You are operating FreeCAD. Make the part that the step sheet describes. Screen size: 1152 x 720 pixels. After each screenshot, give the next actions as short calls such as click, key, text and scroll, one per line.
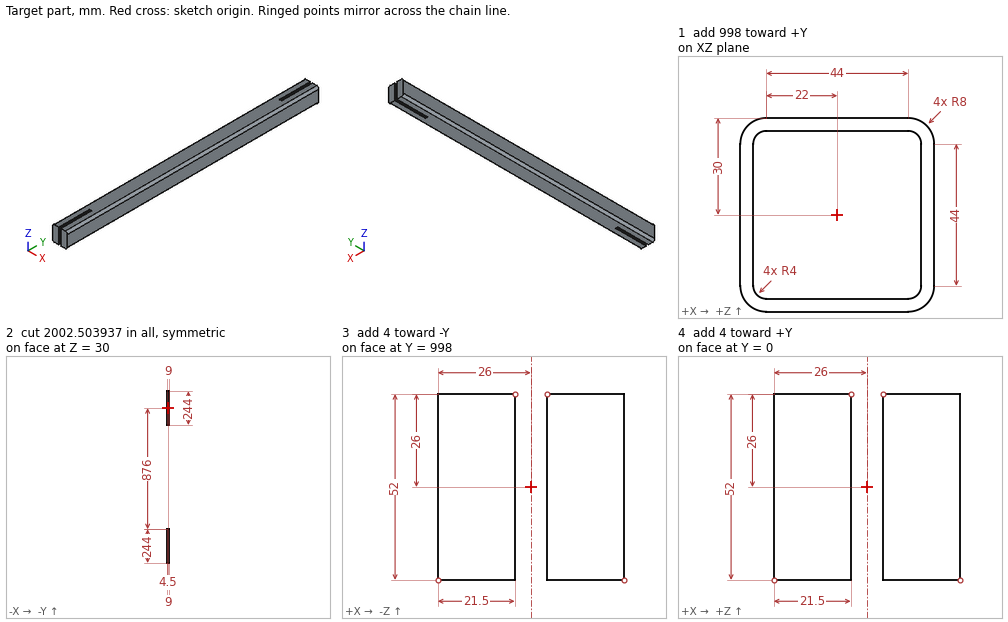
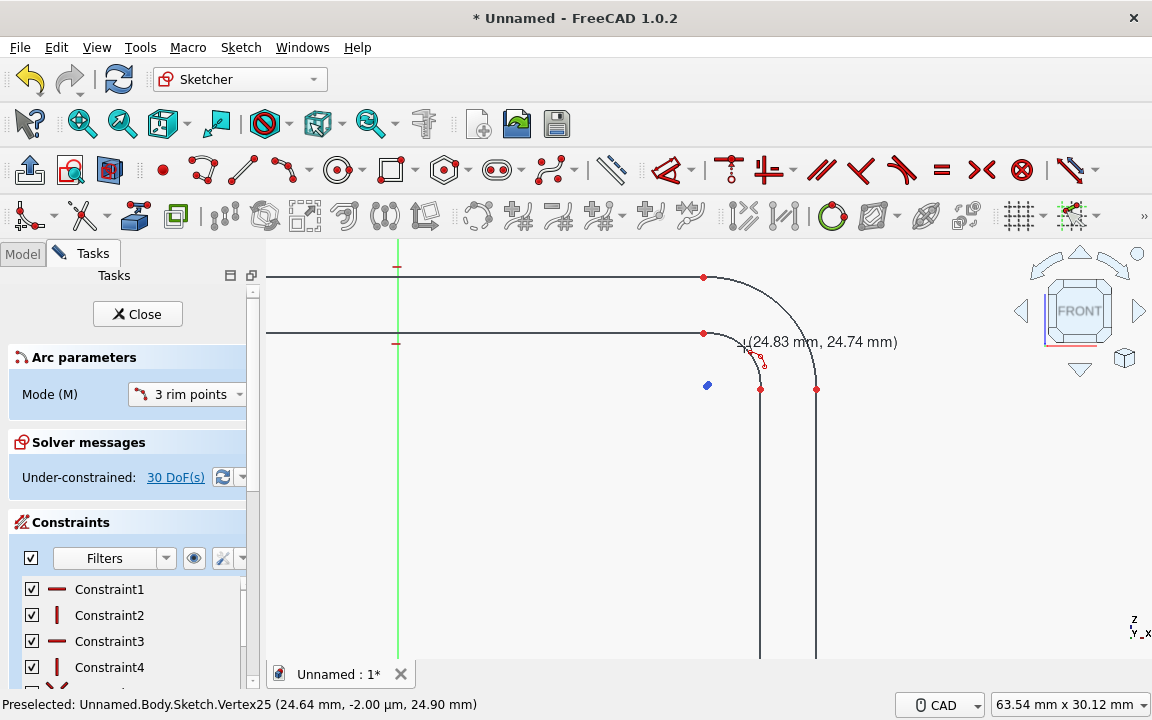
scroll(745, 344, down, 6)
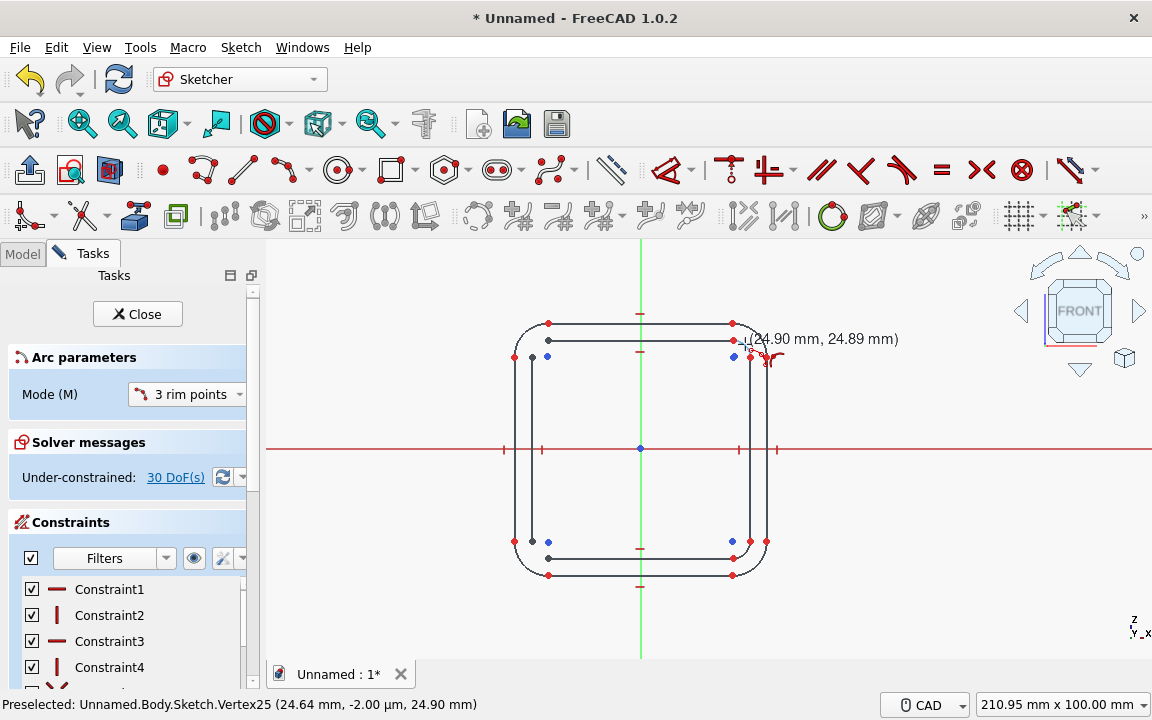
click(548, 341)
click(532, 358)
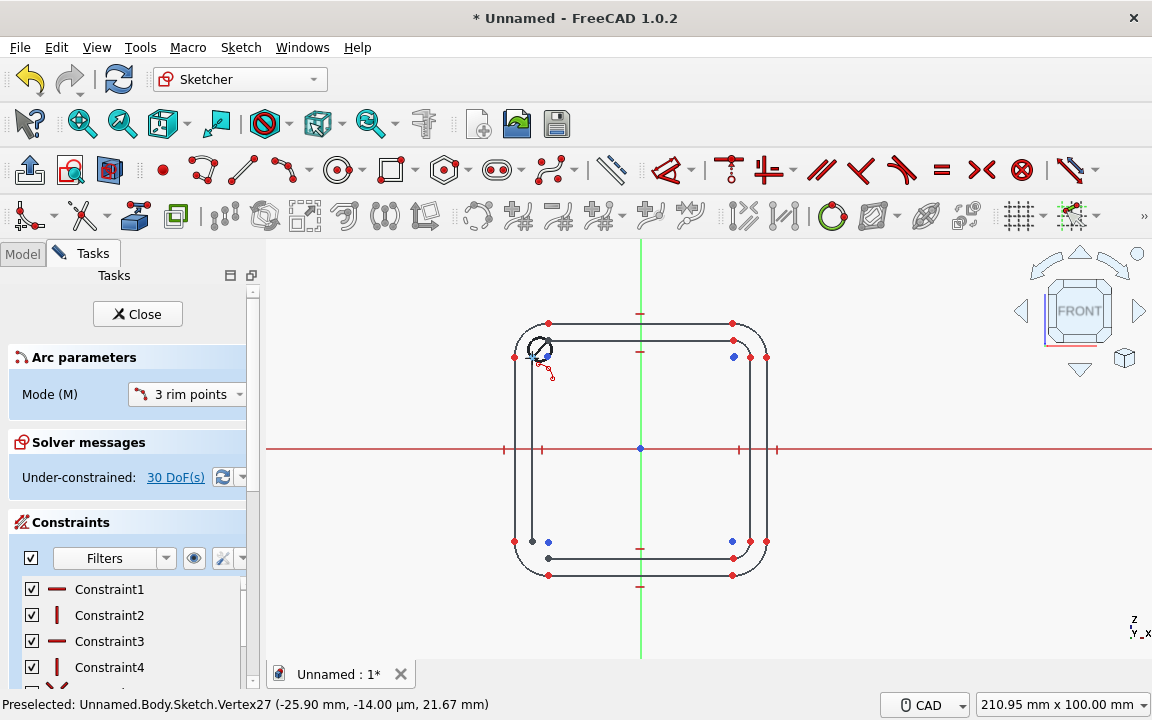
scroll(537, 345, up, 6)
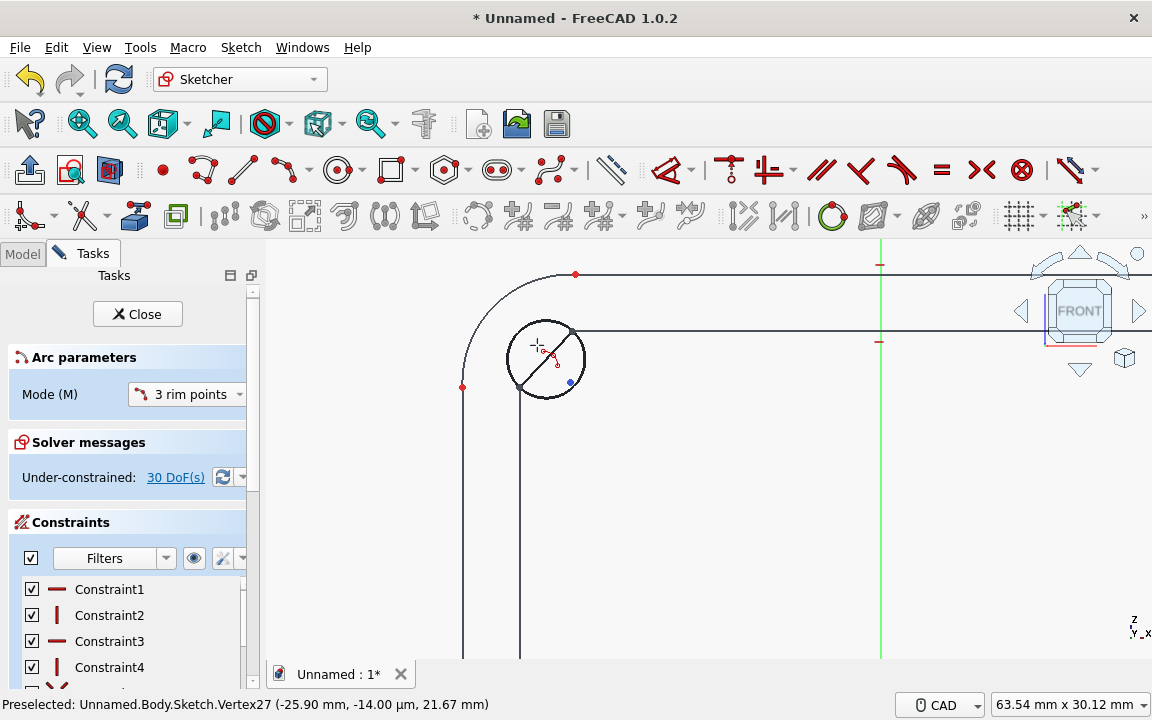
click(535, 343)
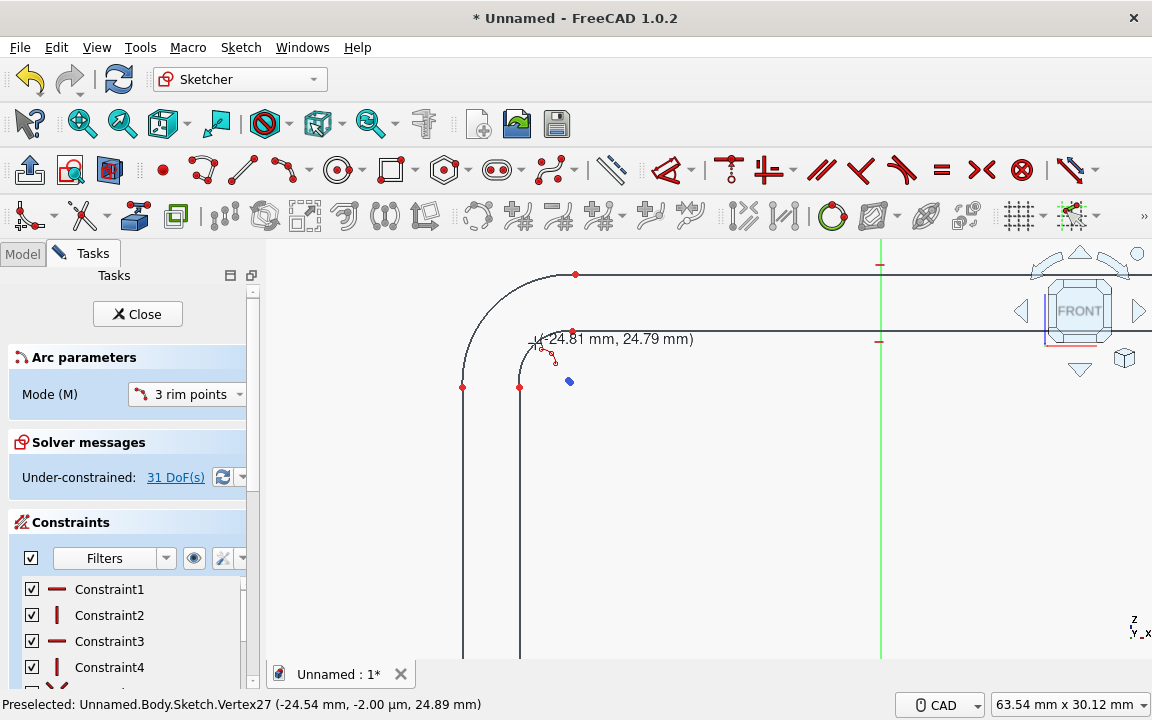
scroll(537, 345, down, 6)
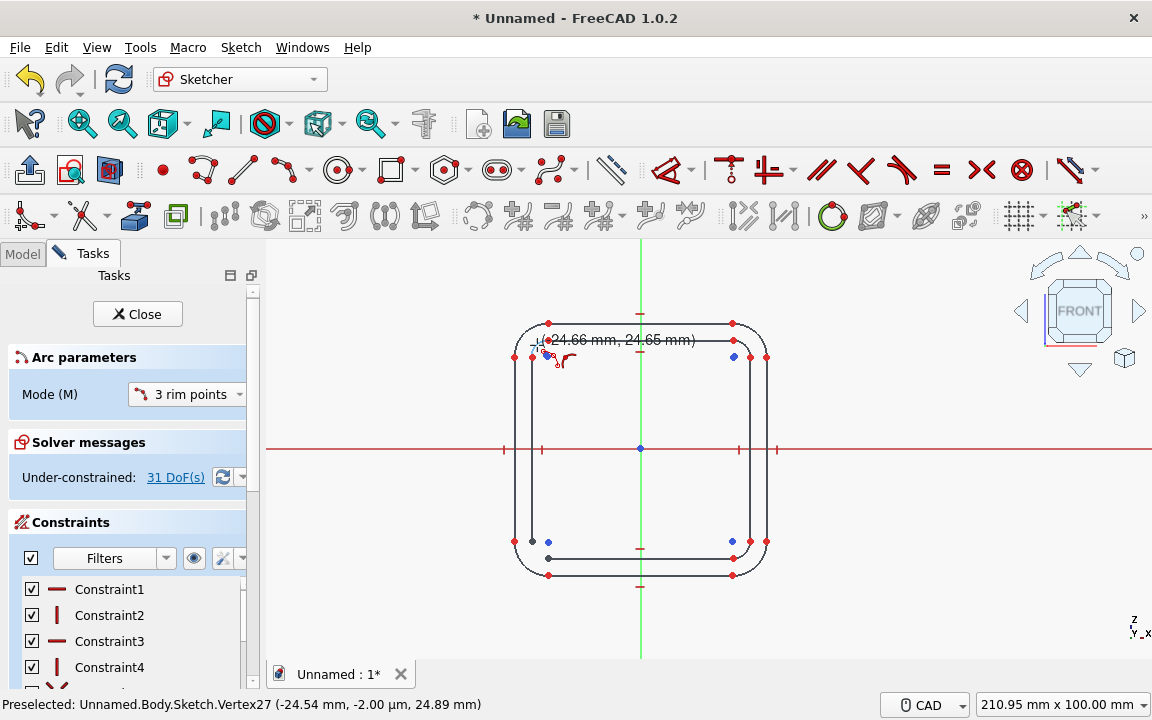
click(532, 542)
click(548, 559)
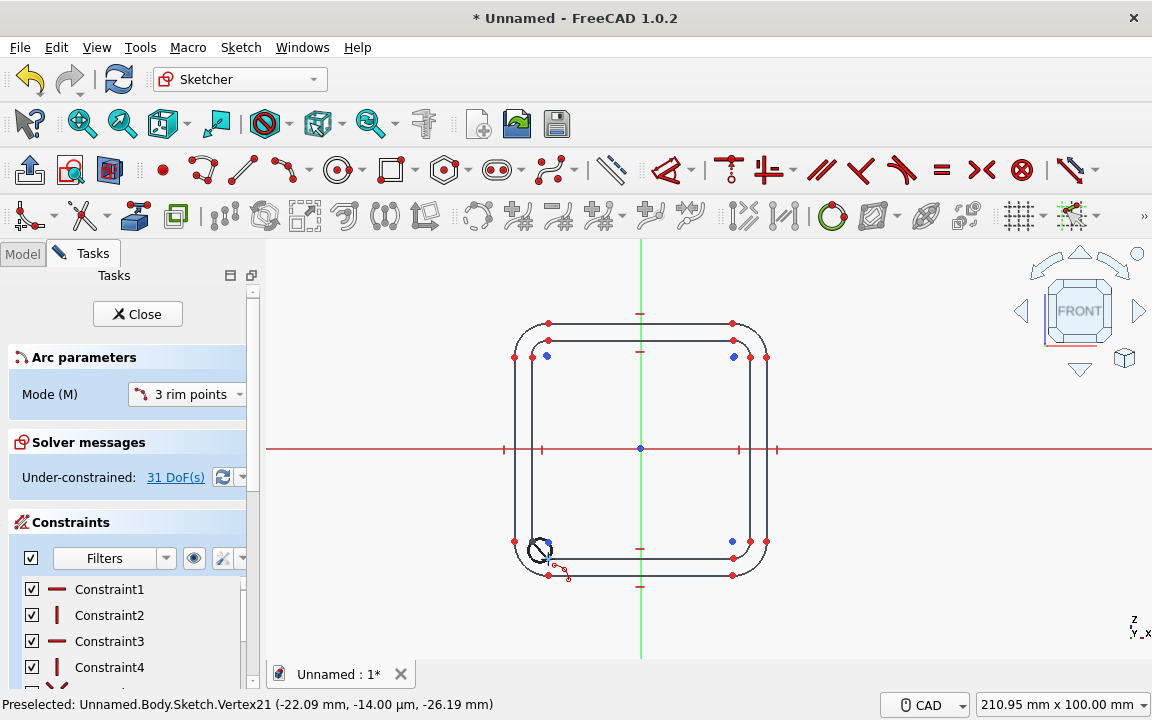
scroll(537, 553, up, 6)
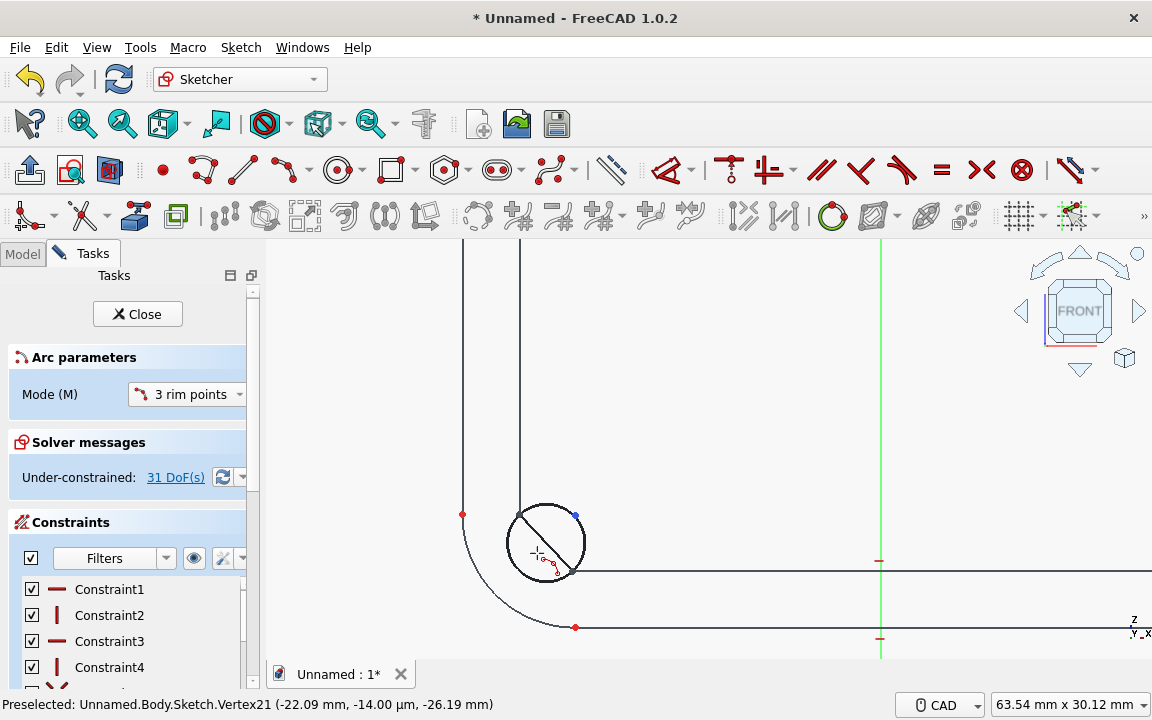
click(535, 552)
key(Escape)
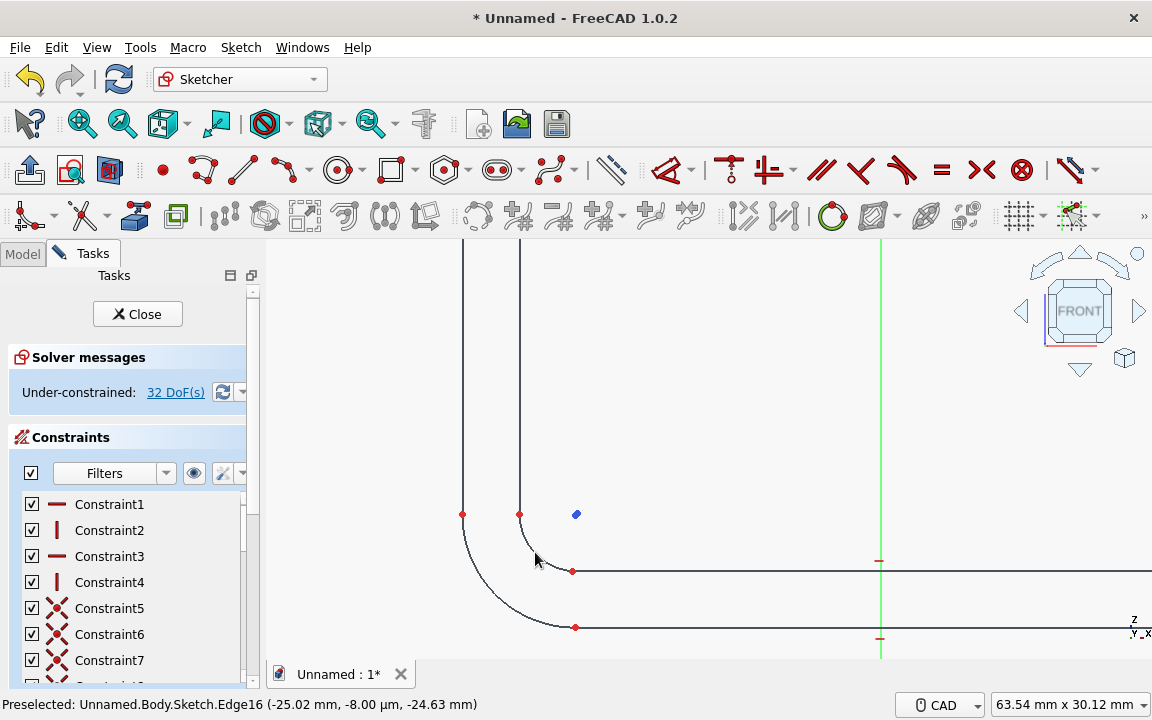
scroll(537, 554, down, 6)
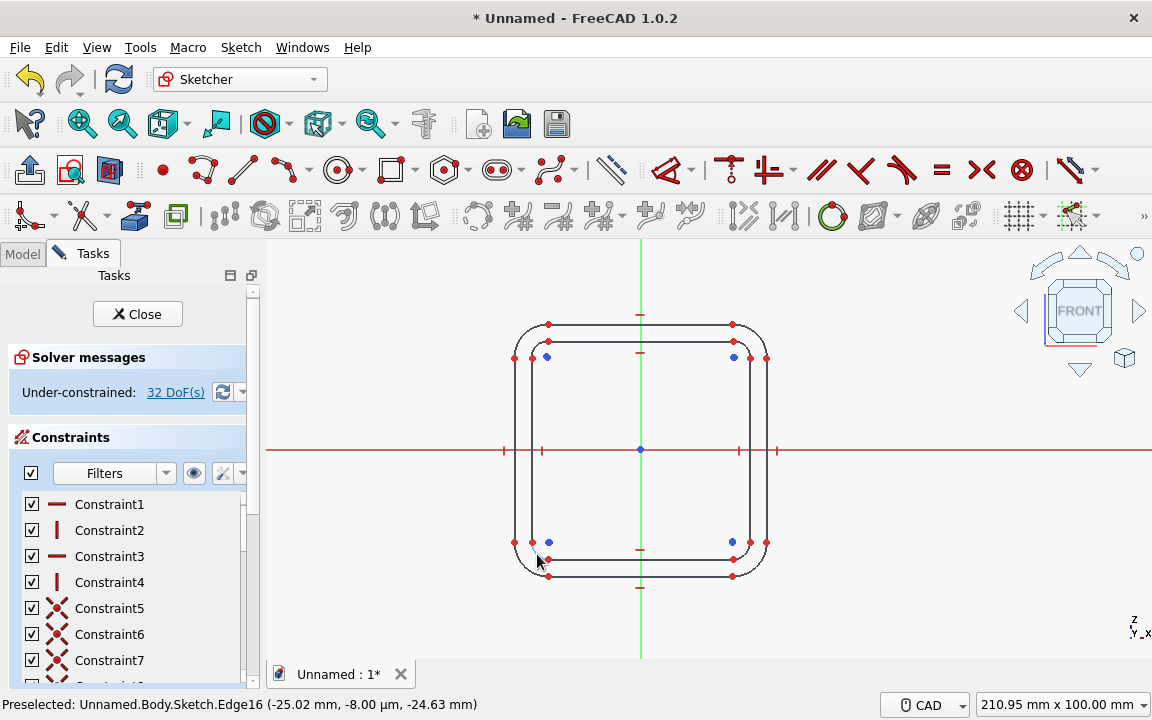
click(604, 325)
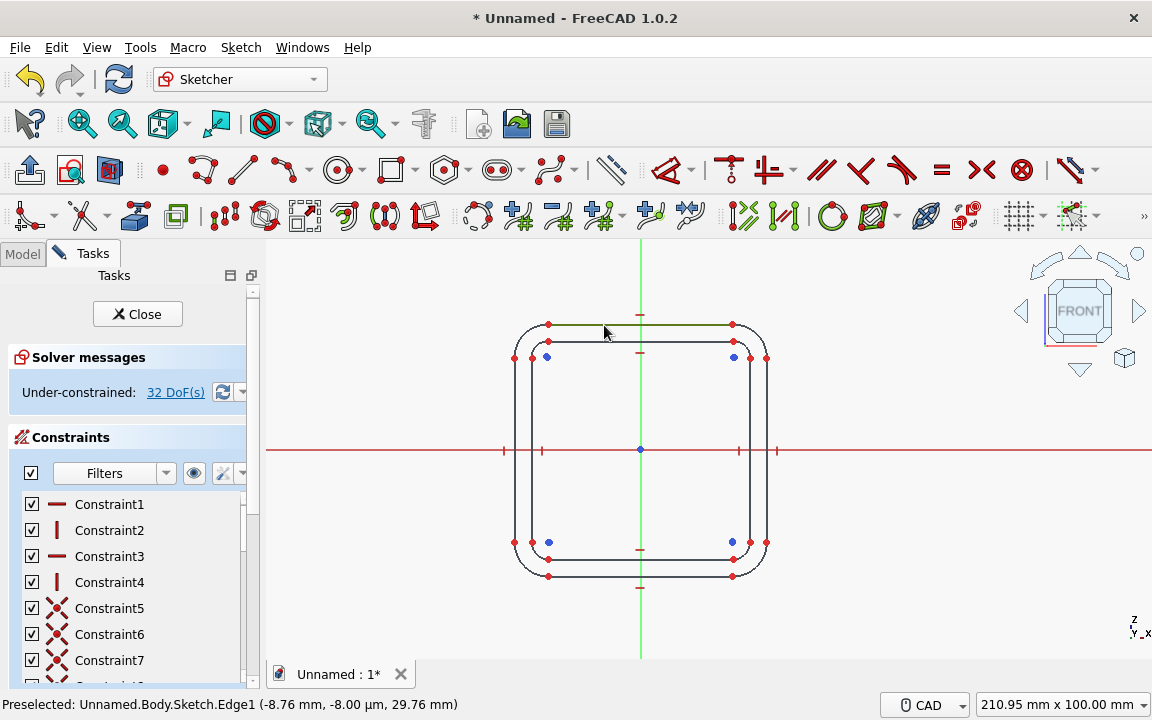
click(763, 343)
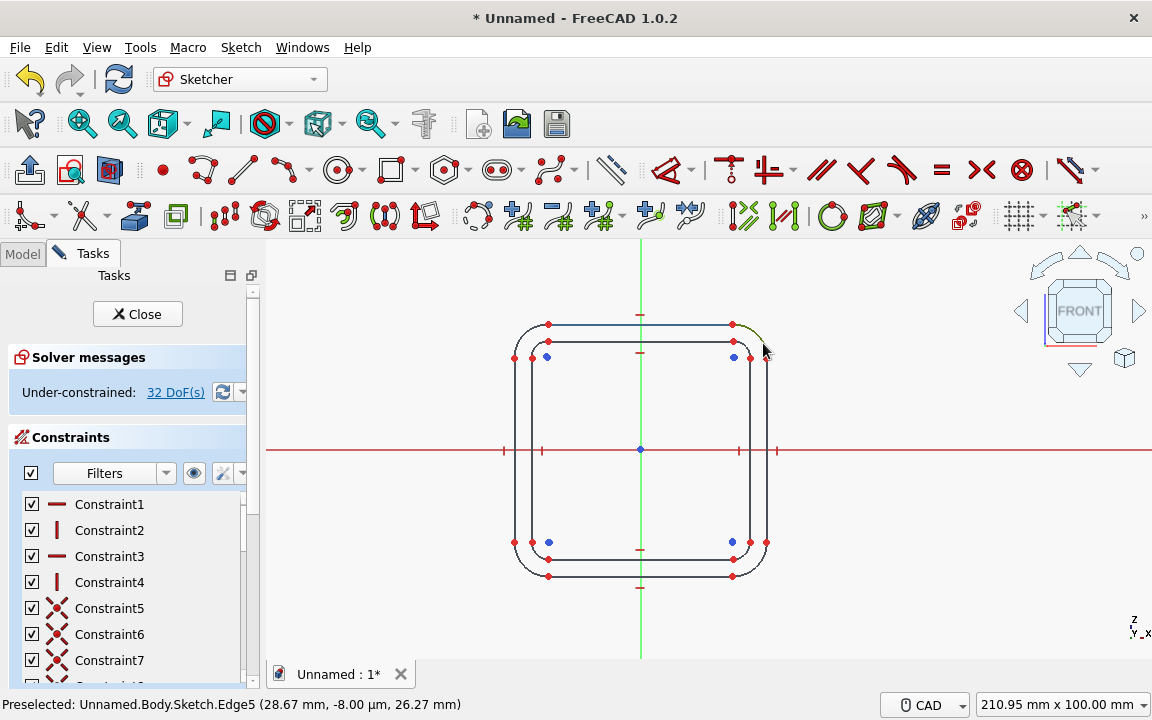
click(902, 170)